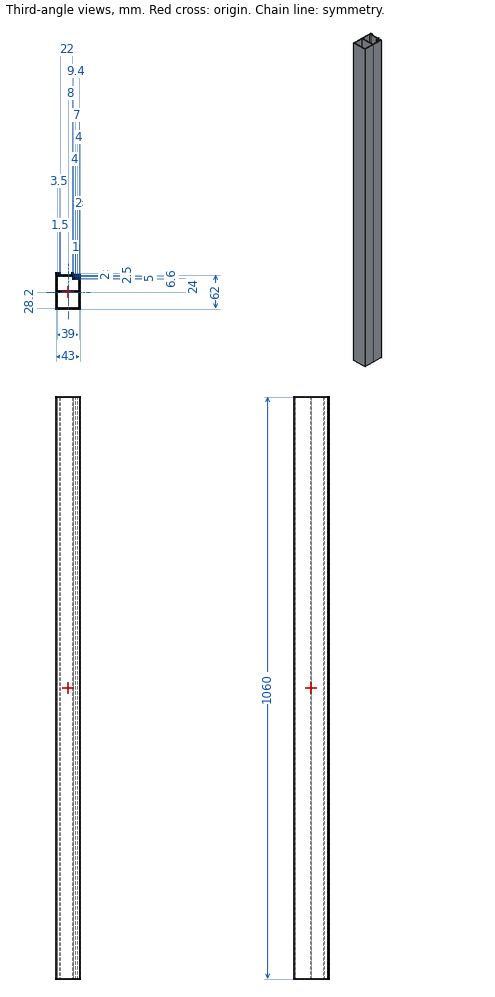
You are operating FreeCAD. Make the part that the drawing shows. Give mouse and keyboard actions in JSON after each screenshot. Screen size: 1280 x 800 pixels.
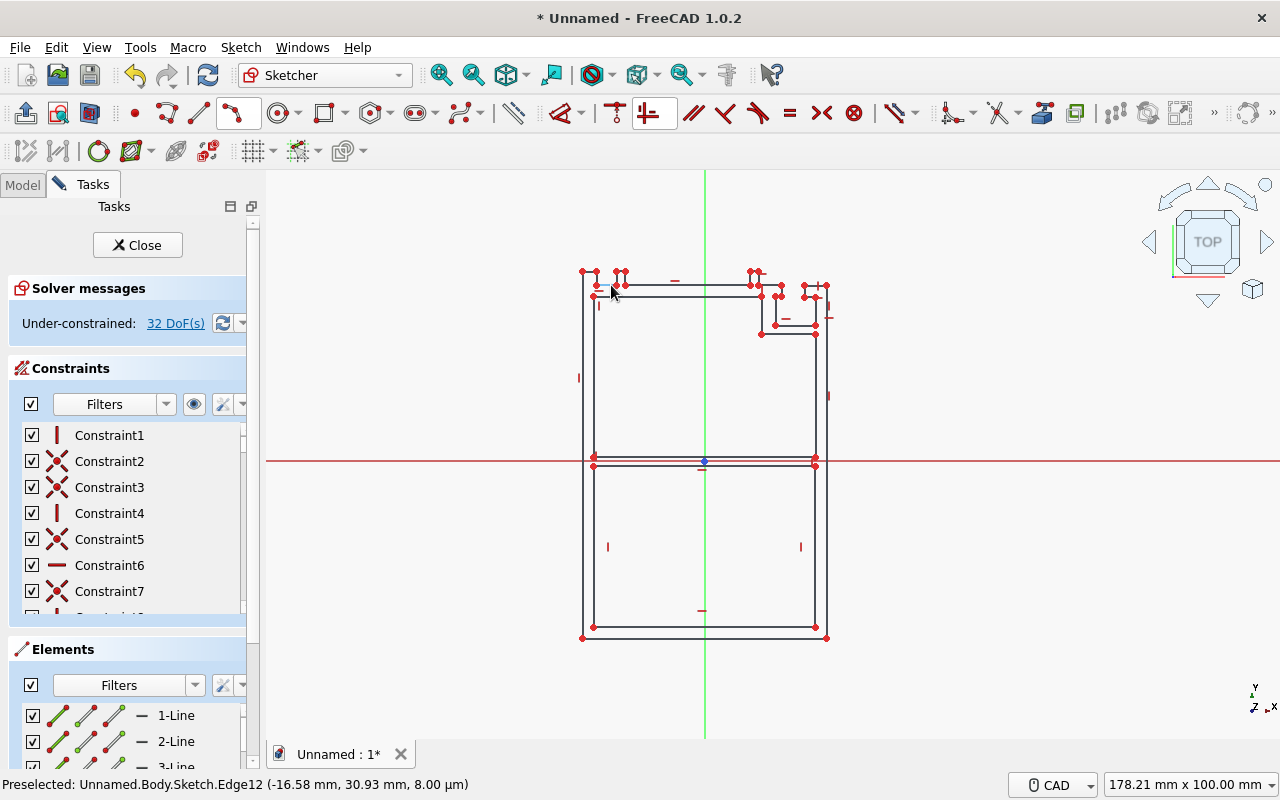
{"action": "left_click", "coordinate": [816, 297]}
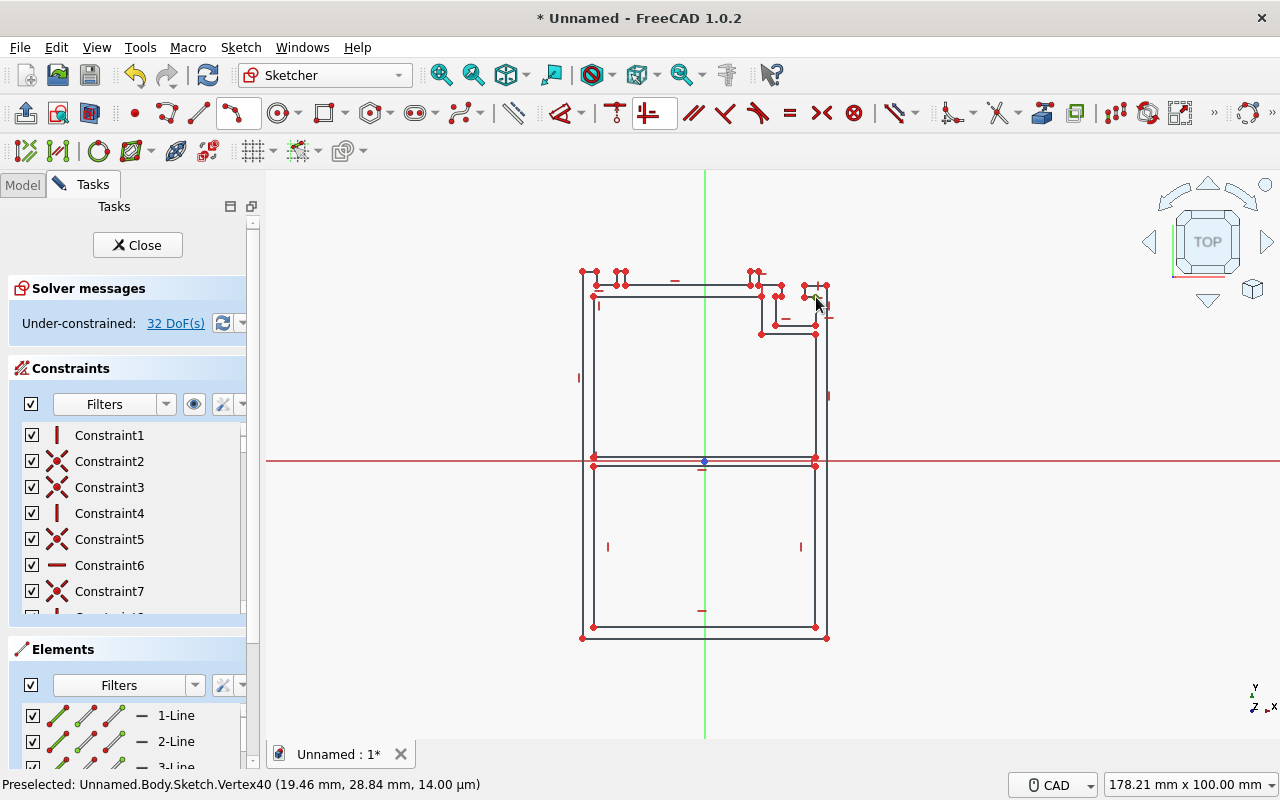
{"action": "left_click", "coordinate": [815, 627]}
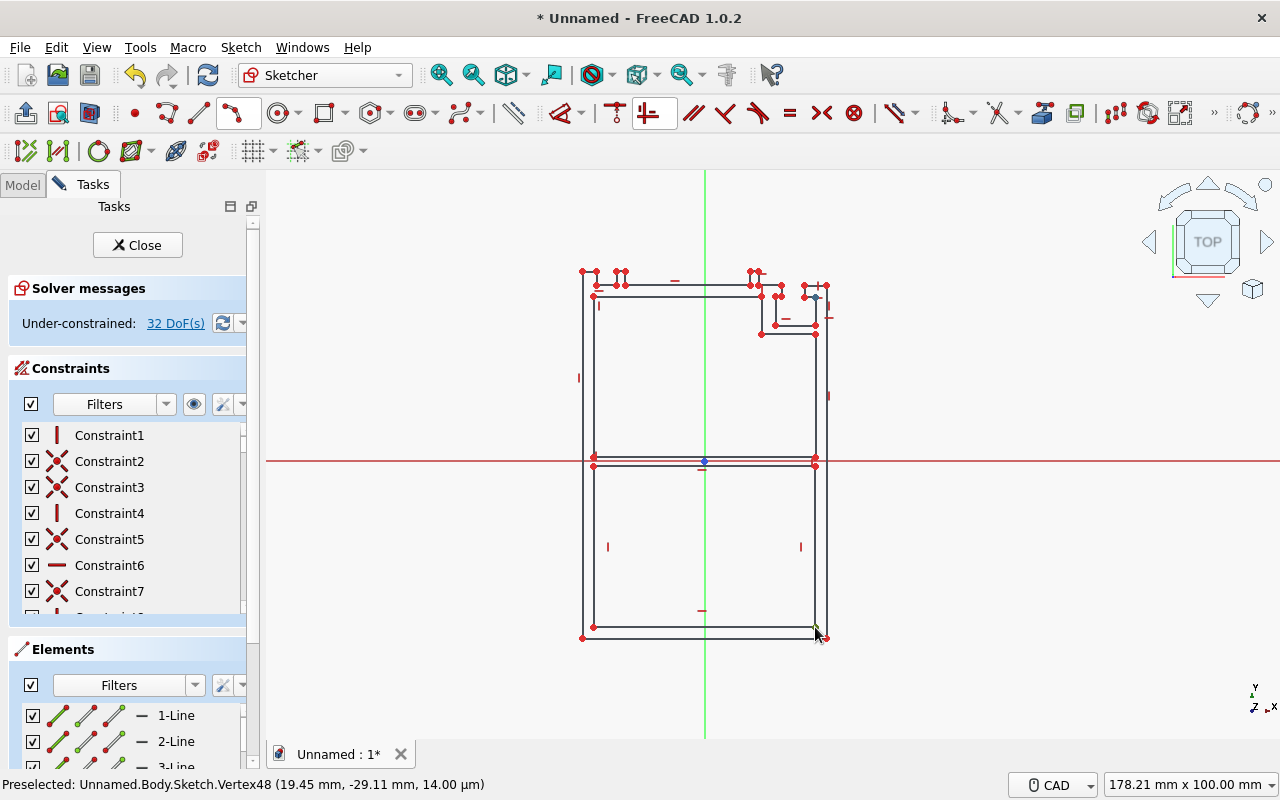
{"action": "left_click", "coordinate": [353, 461]}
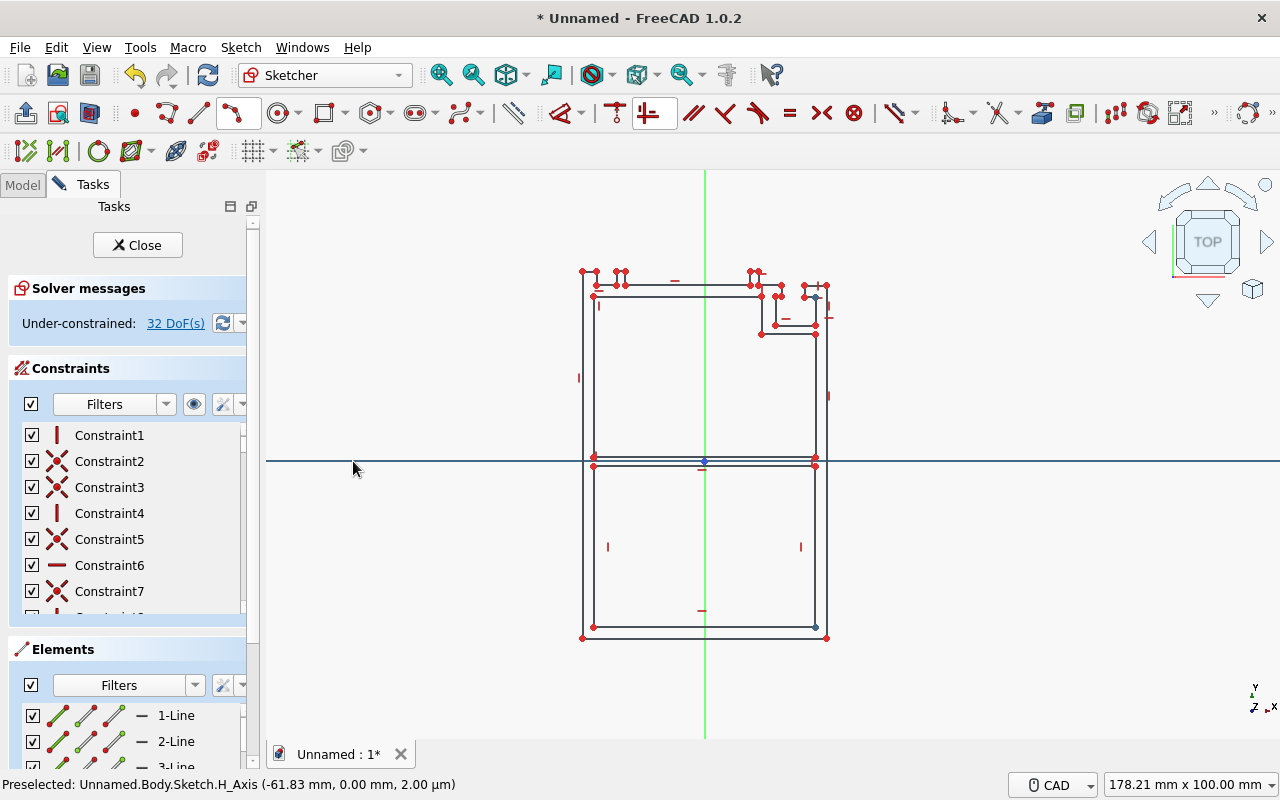
{"action": "left_click", "coordinate": [822, 114]}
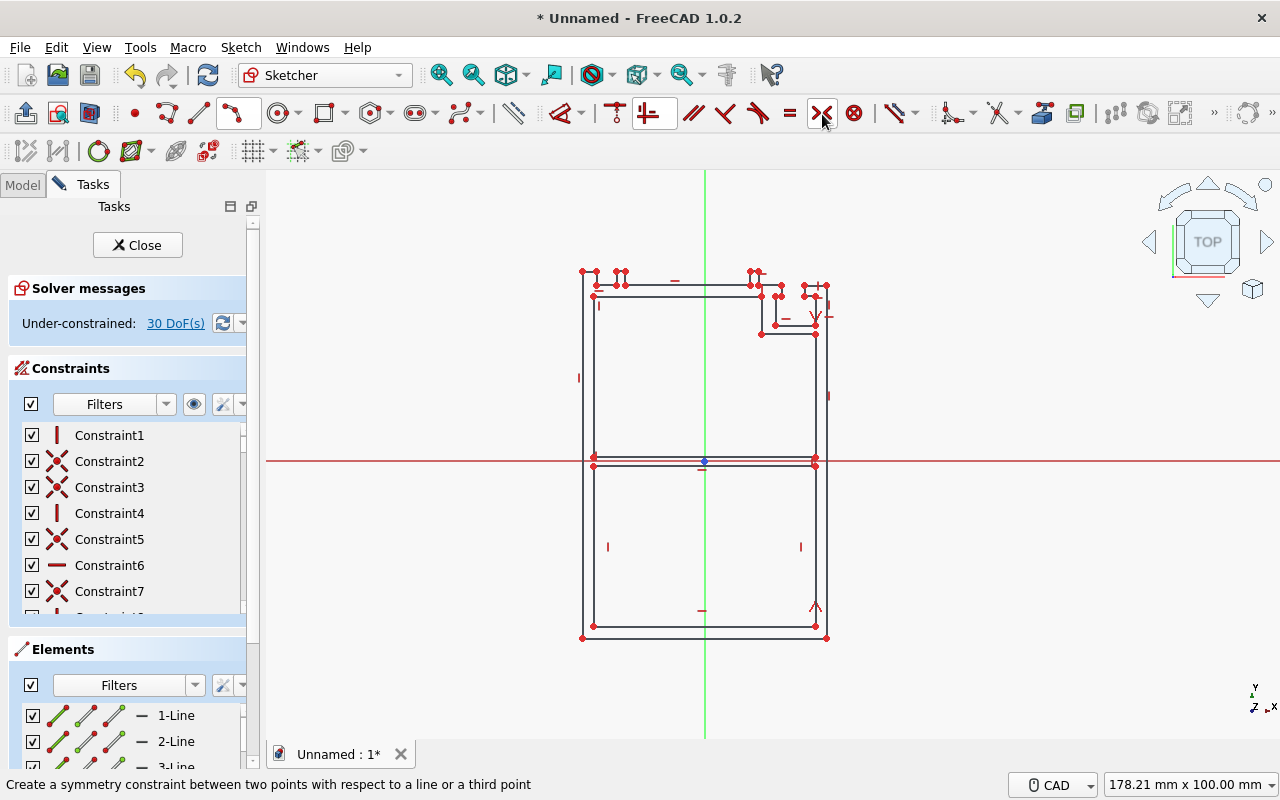
{"action": "scroll", "coordinate": [816, 466], "scroll_direction": "up", "scroll_amount": 2}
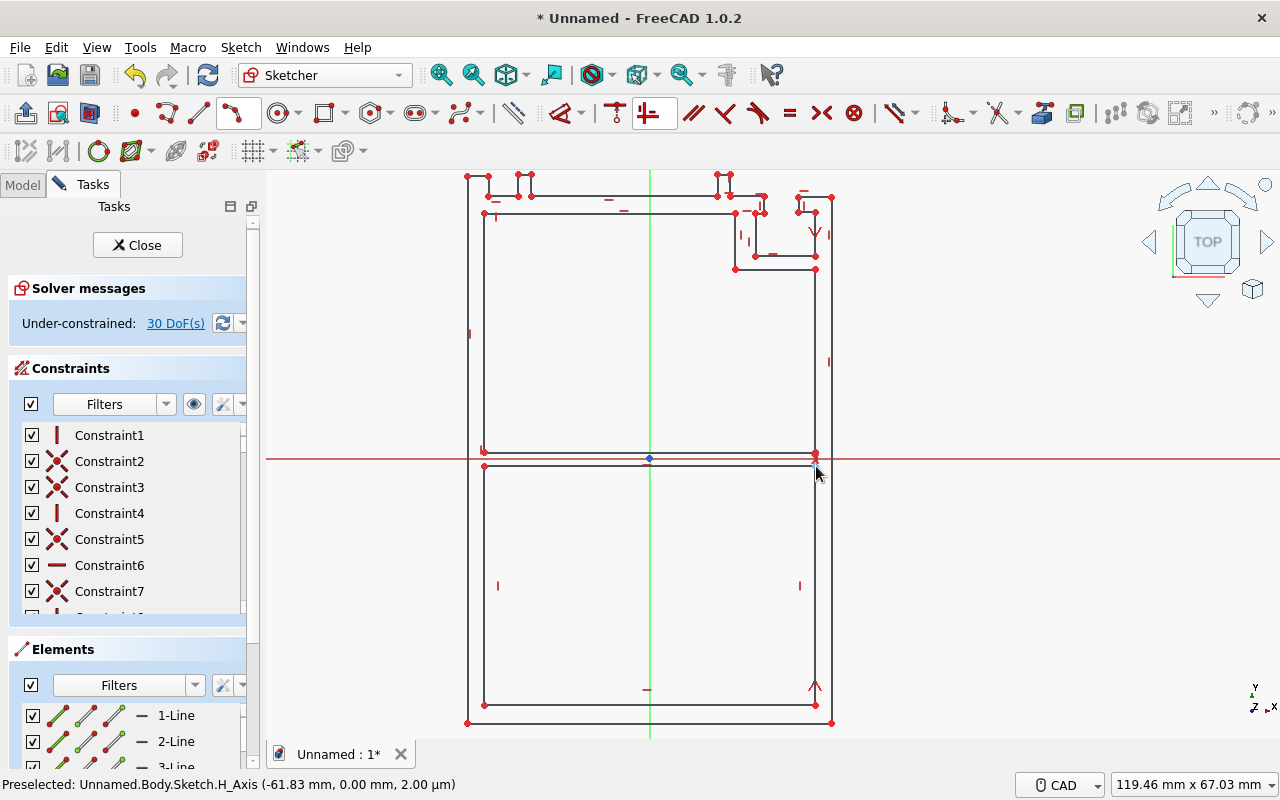
{"action": "left_click", "coordinate": [815, 466]}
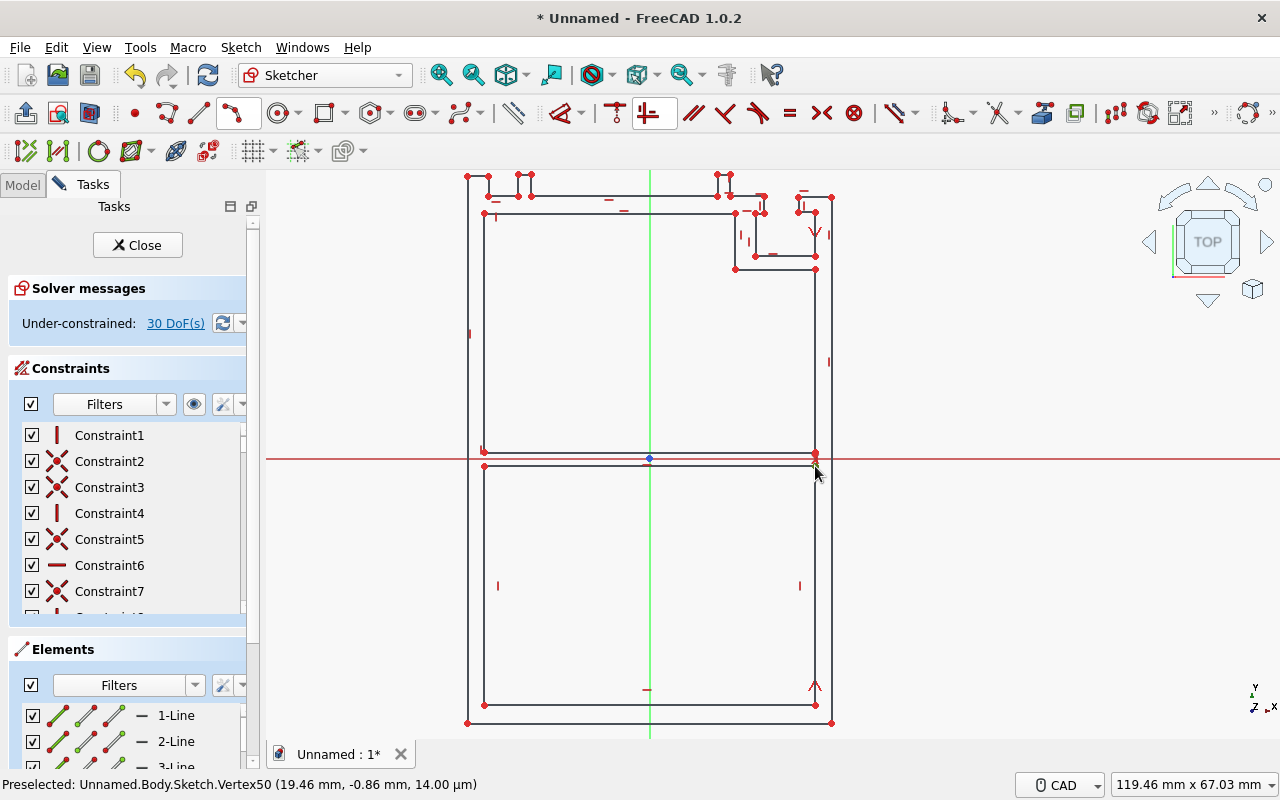
{"action": "left_click", "coordinate": [815, 453]}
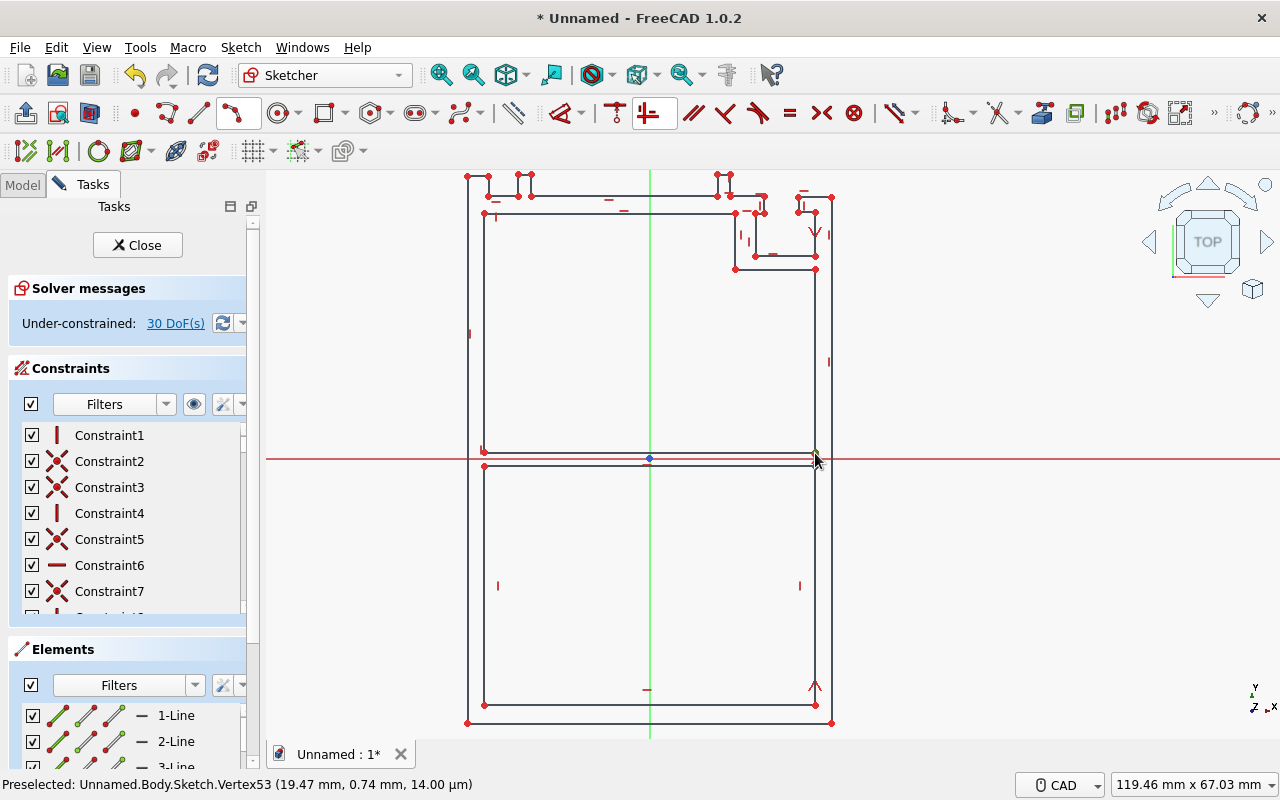
{"action": "left_click", "coordinate": [353, 459]}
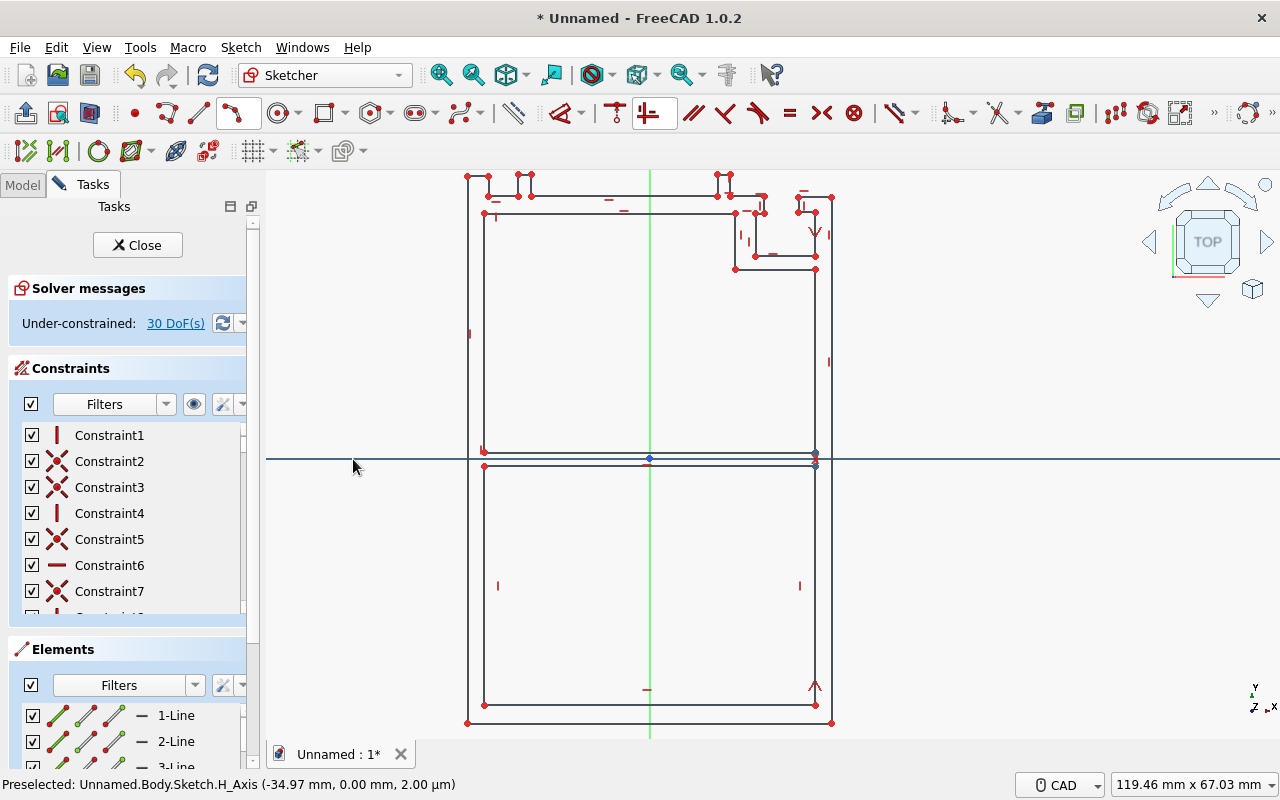
{"action": "left_click", "coordinate": [822, 114]}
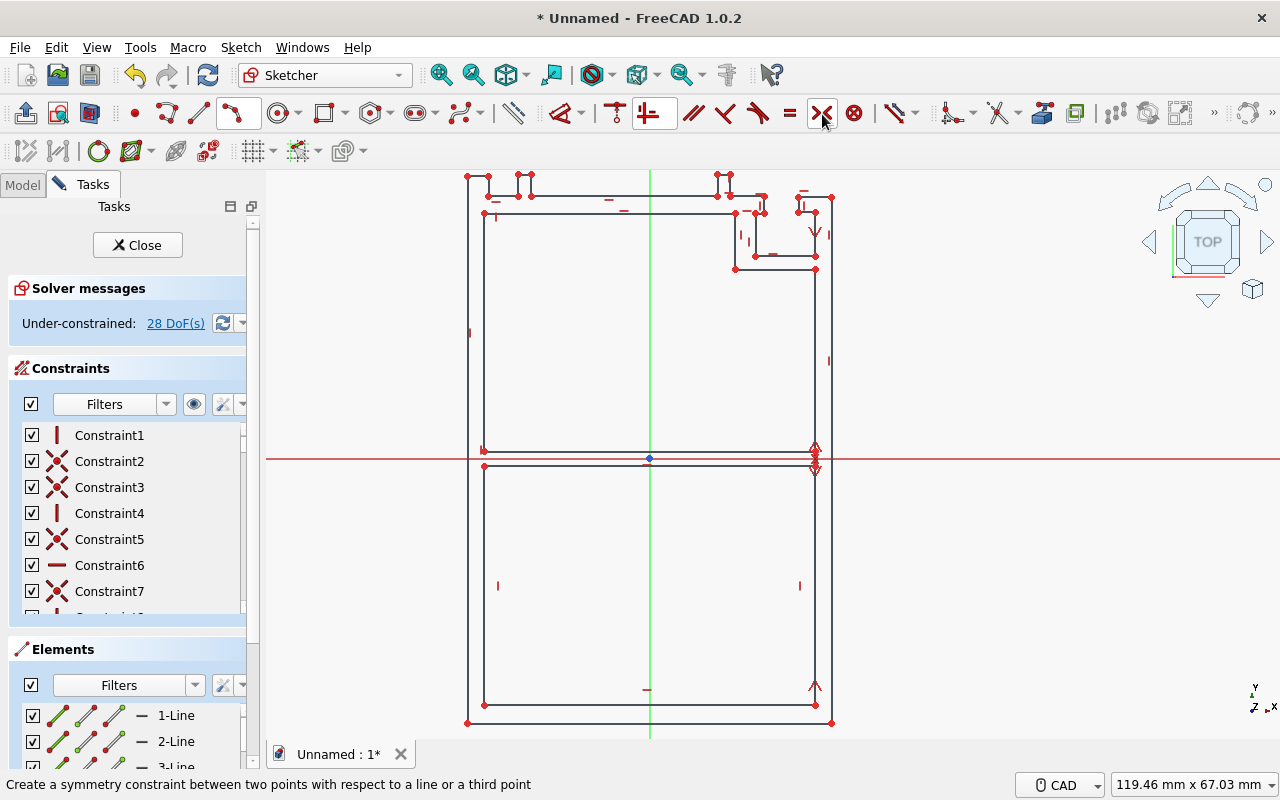
{"action": "left_click", "coordinate": [815, 212]}